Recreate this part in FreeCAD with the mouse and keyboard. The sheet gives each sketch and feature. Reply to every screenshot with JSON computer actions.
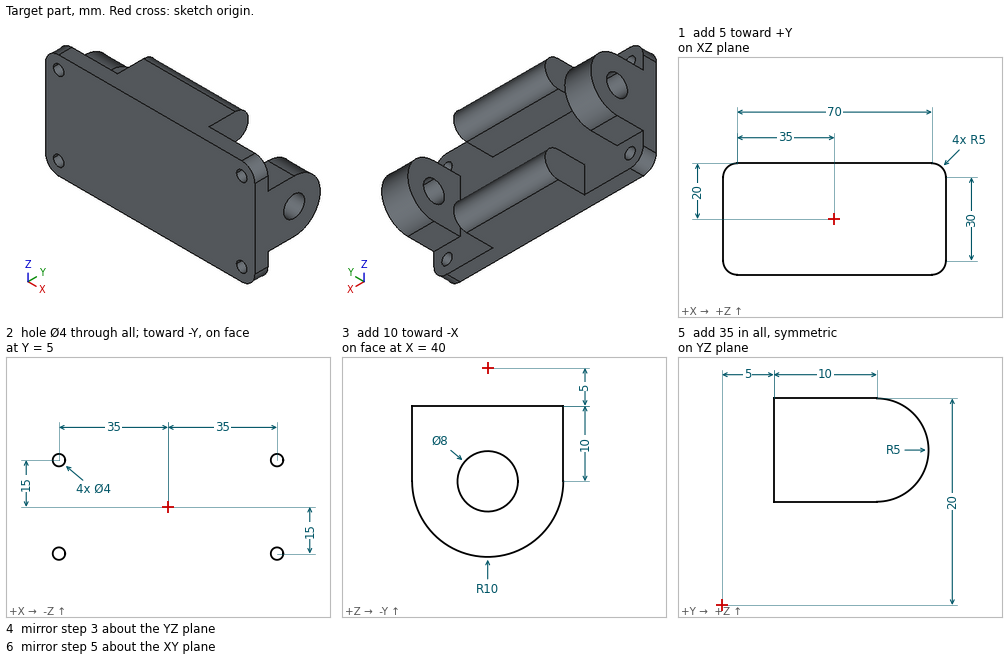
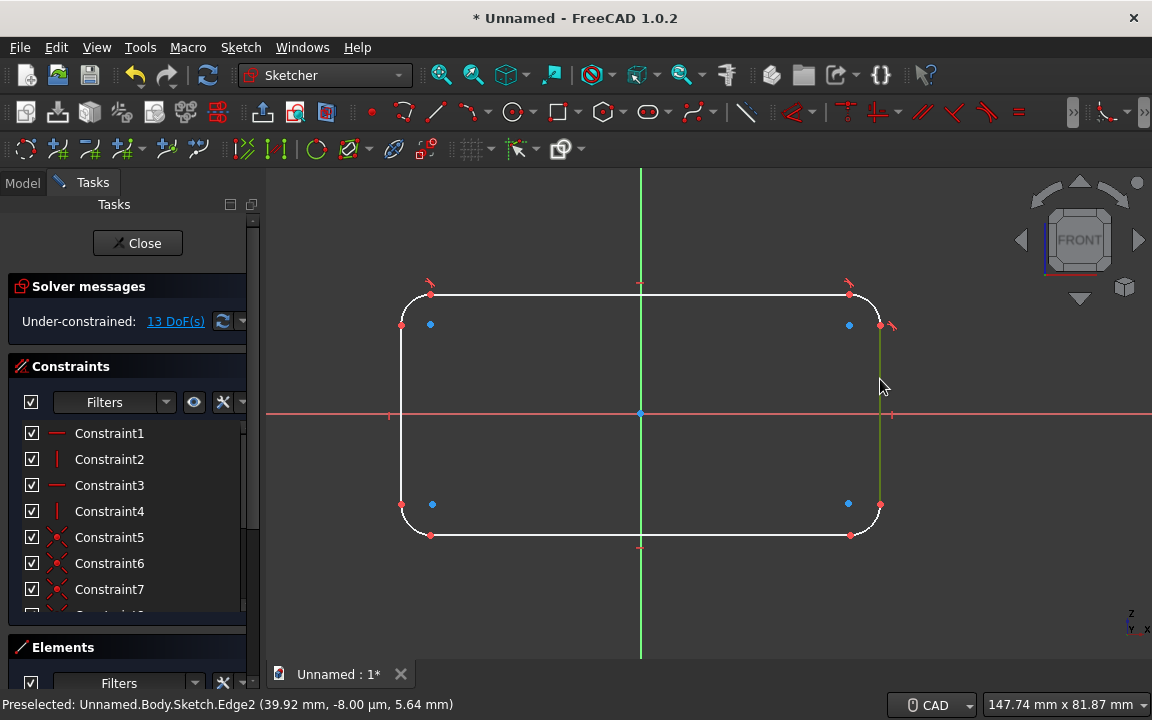
{"action": "left_click", "coordinate": [864, 531]}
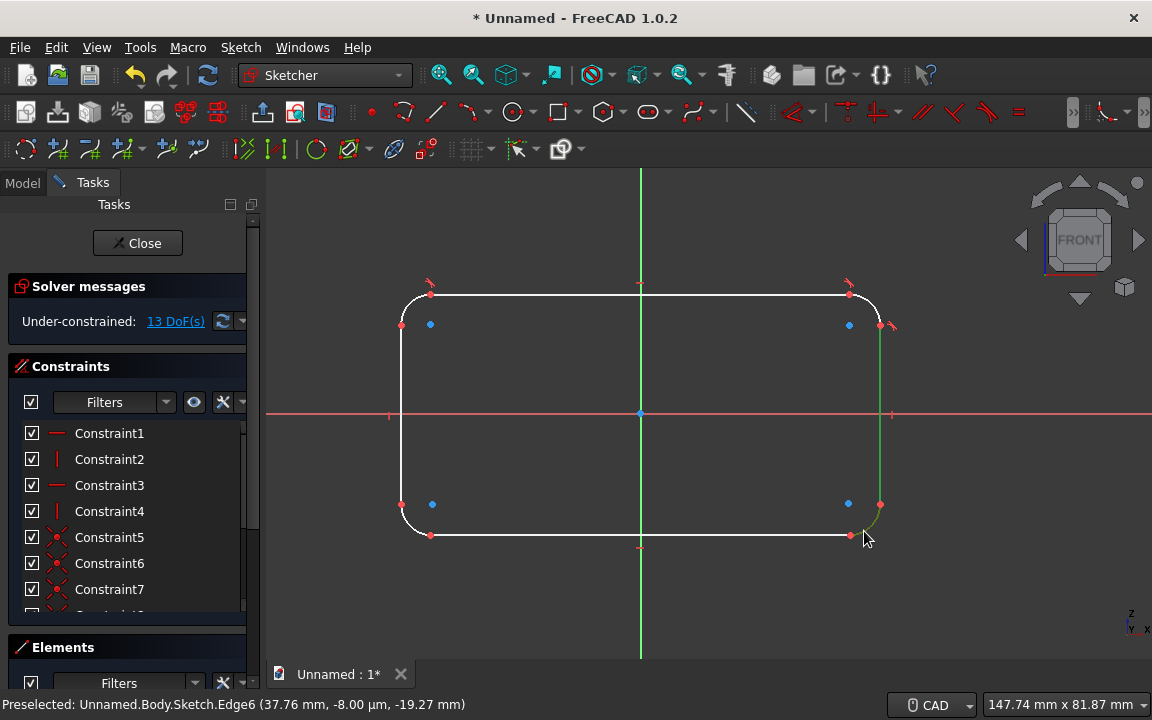
{"action": "left_click", "coordinate": [988, 112]}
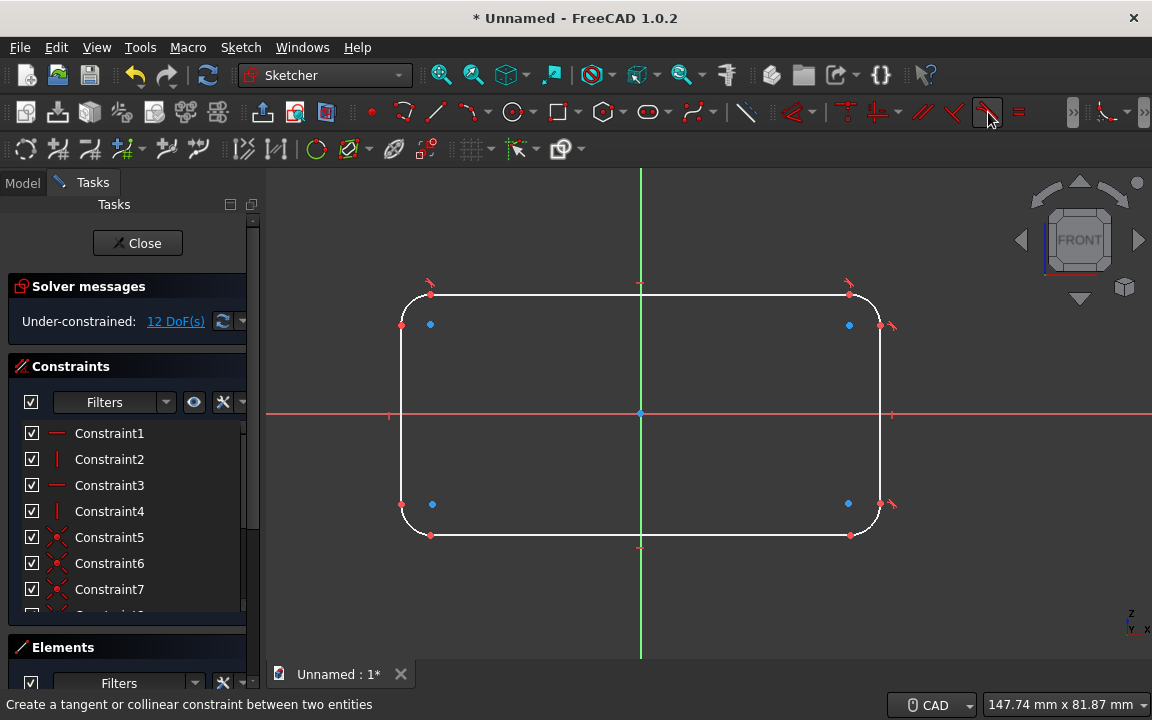
{"action": "left_click", "coordinate": [725, 535]}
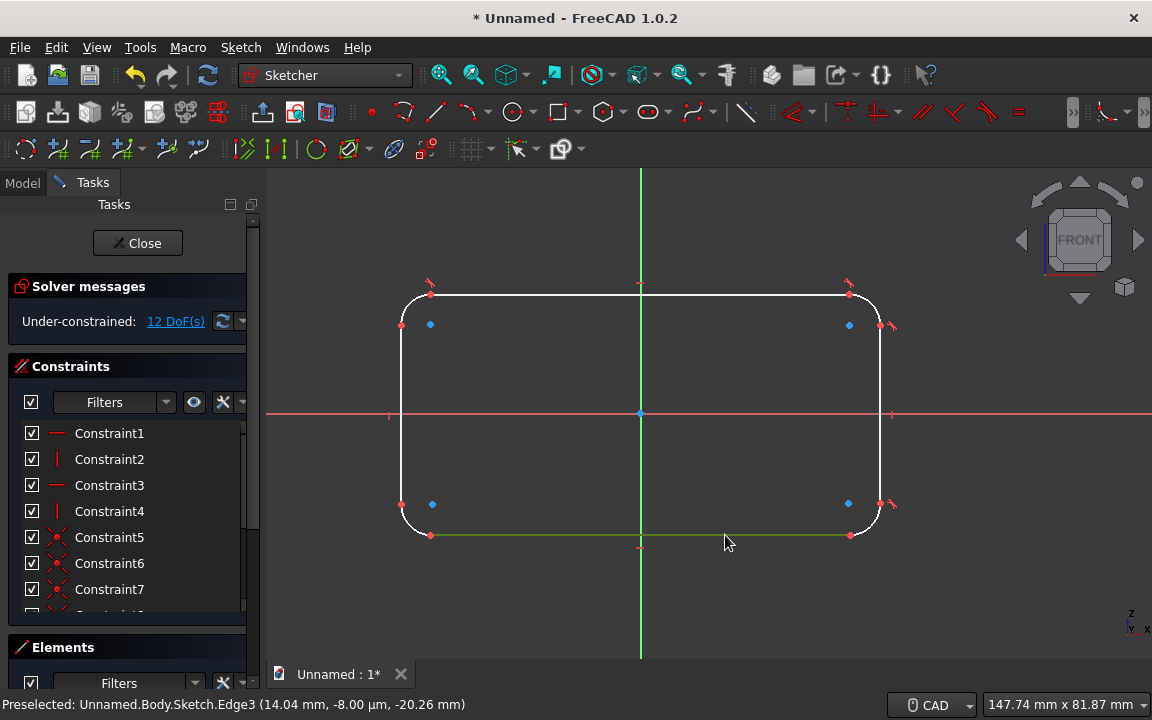
{"action": "left_click", "coordinate": [864, 531]}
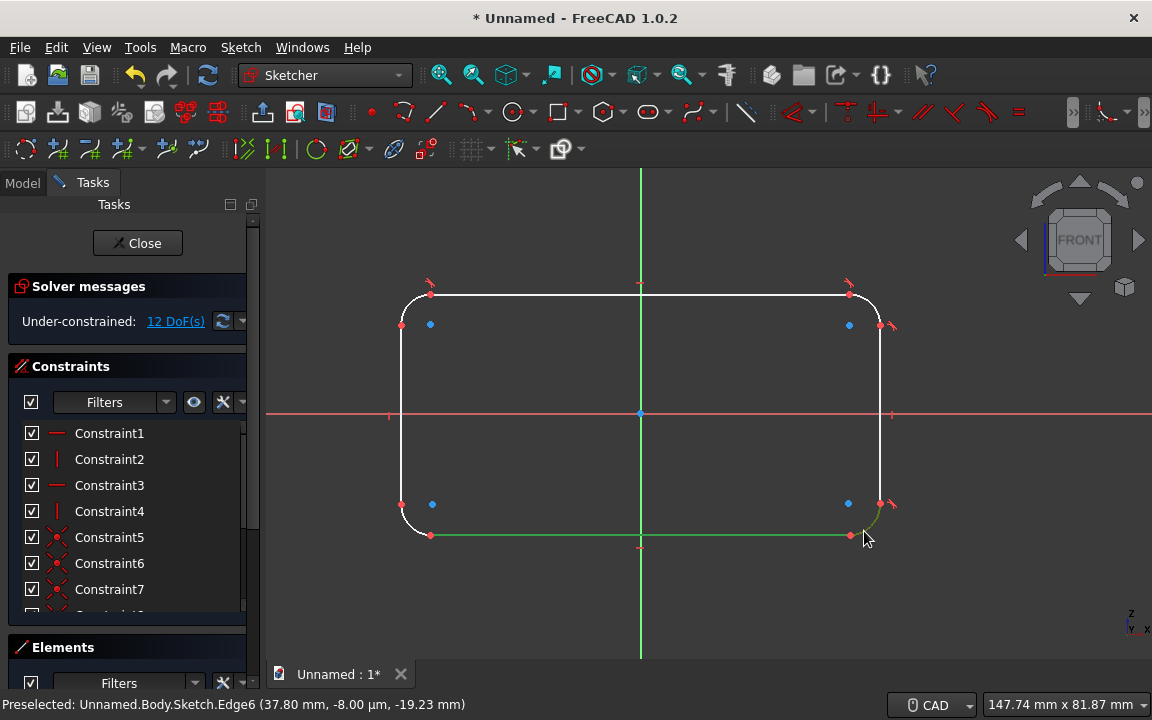
{"action": "left_click", "coordinate": [988, 112]}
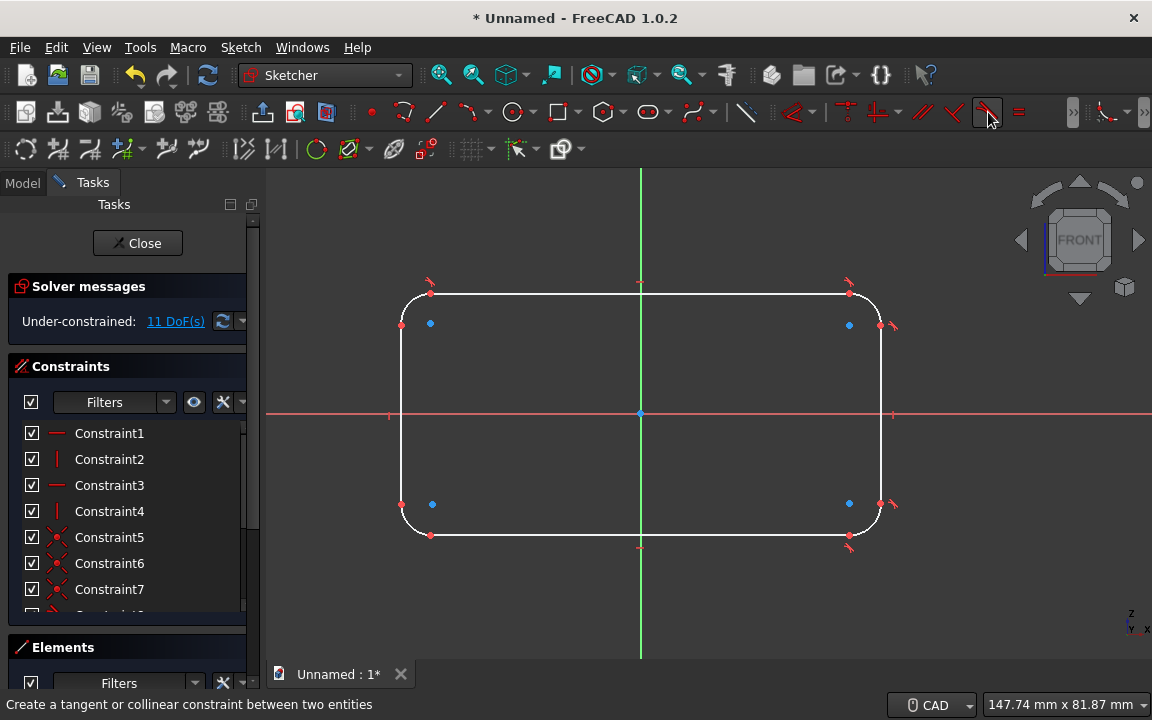
{"action": "left_click", "coordinate": [724, 535]}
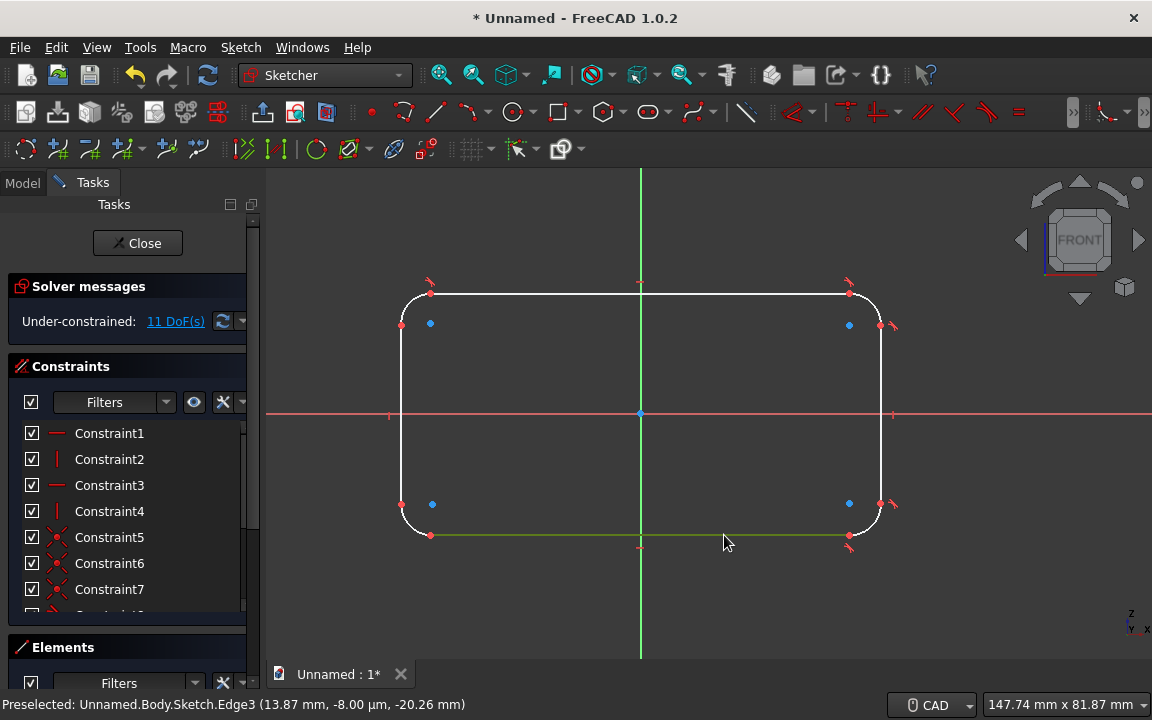
{"action": "left_click", "coordinate": [405, 518]}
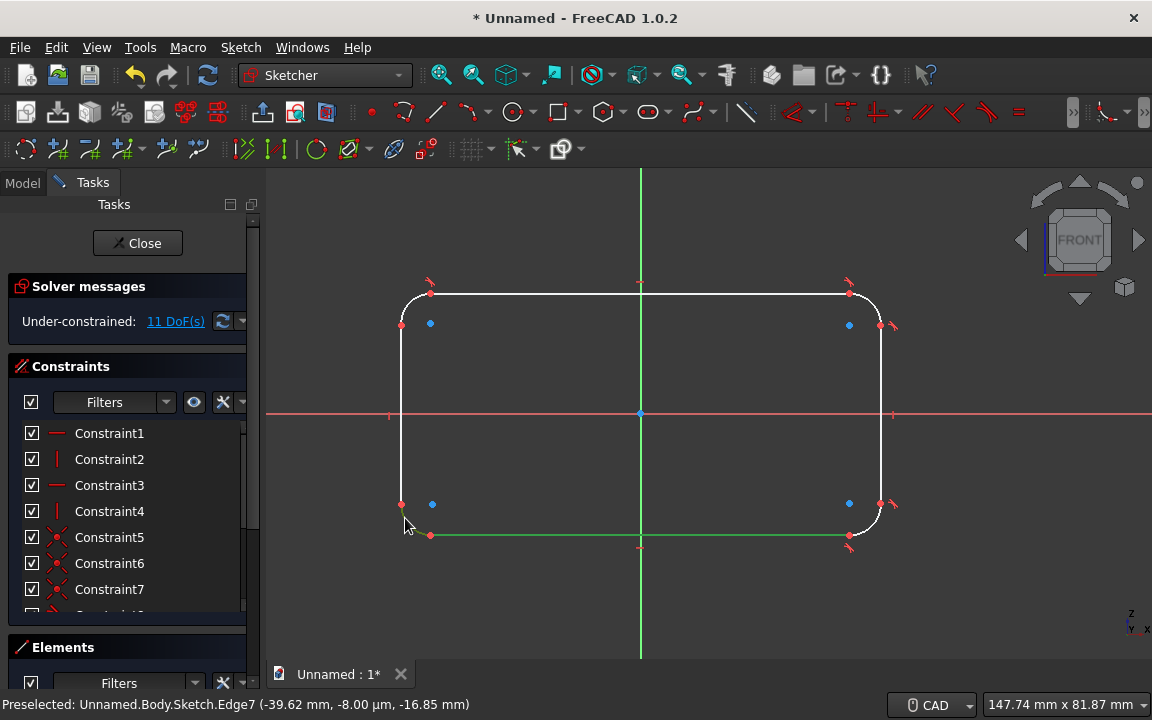
{"action": "key", "text": "t"}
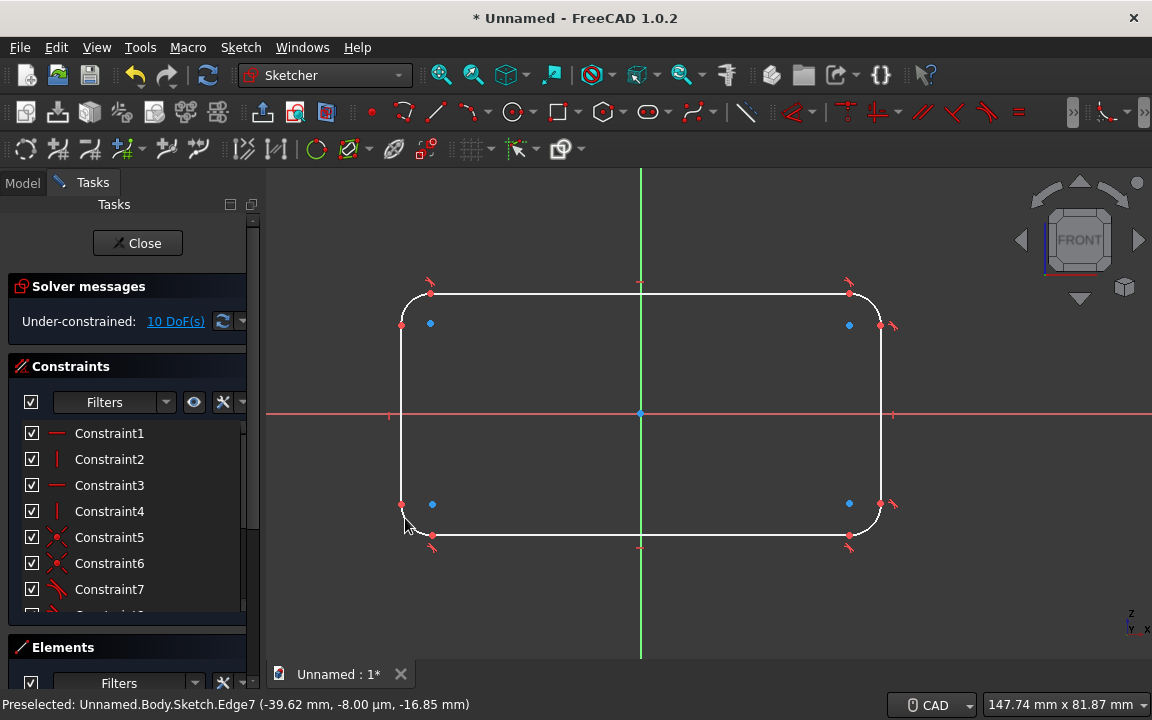
{"action": "left_click", "coordinate": [401, 451]}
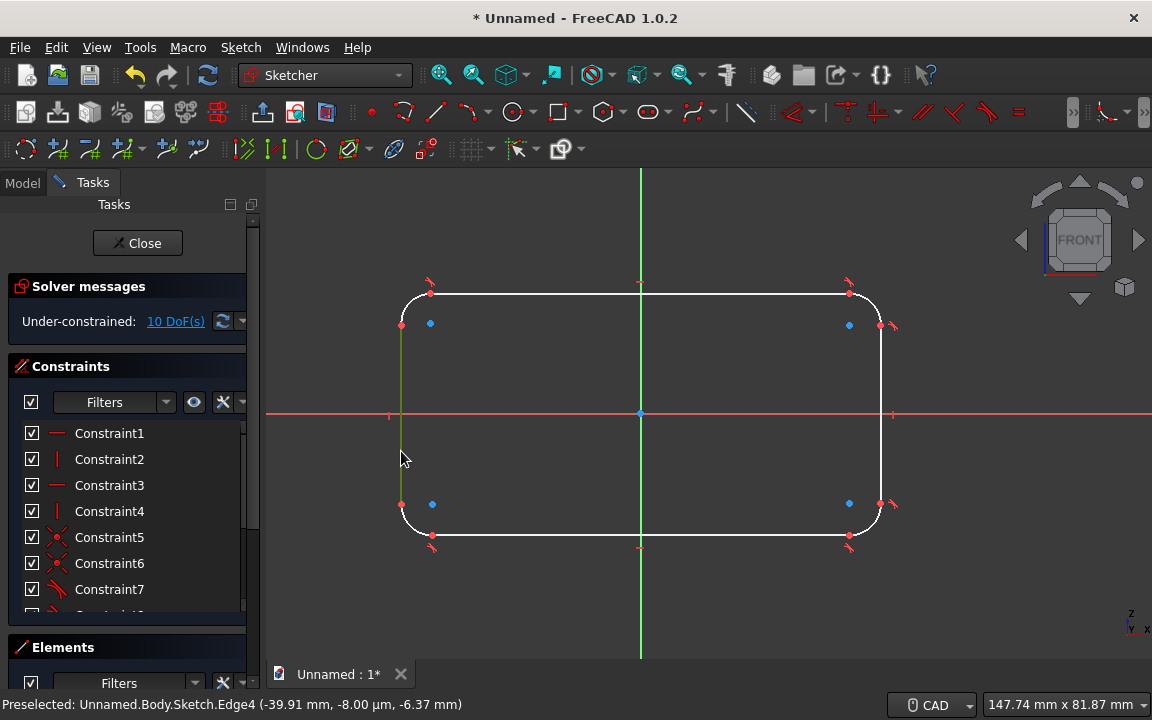
{"action": "left_click", "coordinate": [405, 519]}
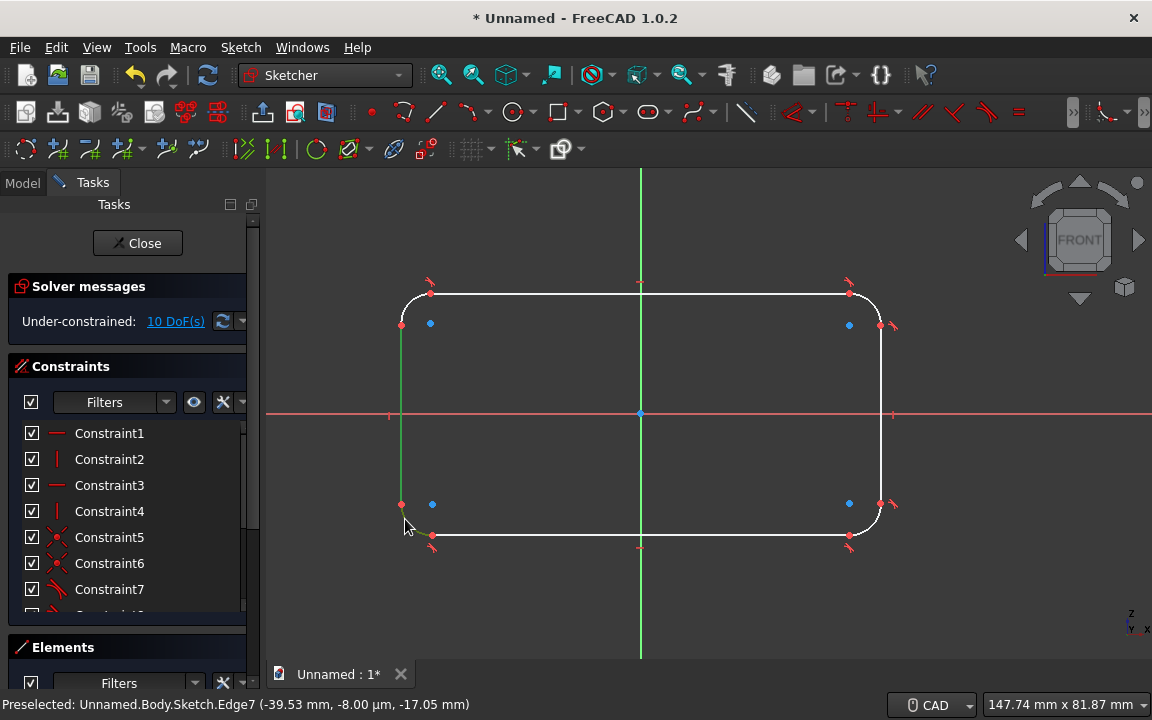
{"action": "left_click", "coordinate": [988, 112]}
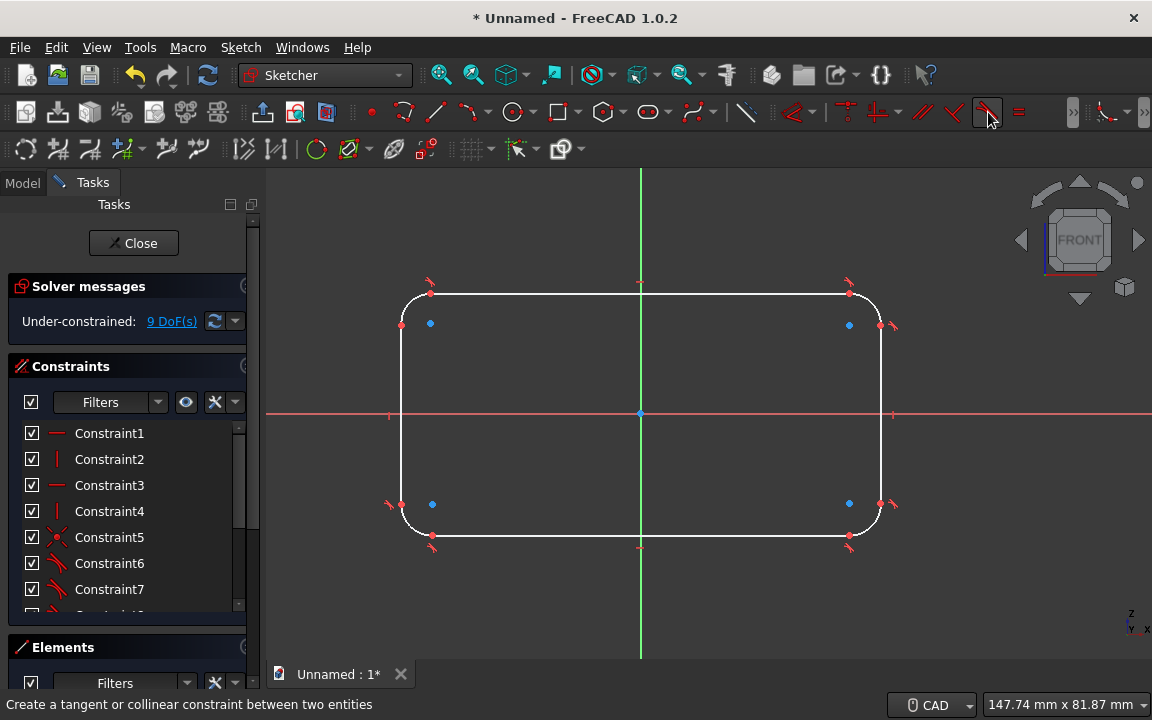
{"action": "left_click", "coordinate": [401, 451]}